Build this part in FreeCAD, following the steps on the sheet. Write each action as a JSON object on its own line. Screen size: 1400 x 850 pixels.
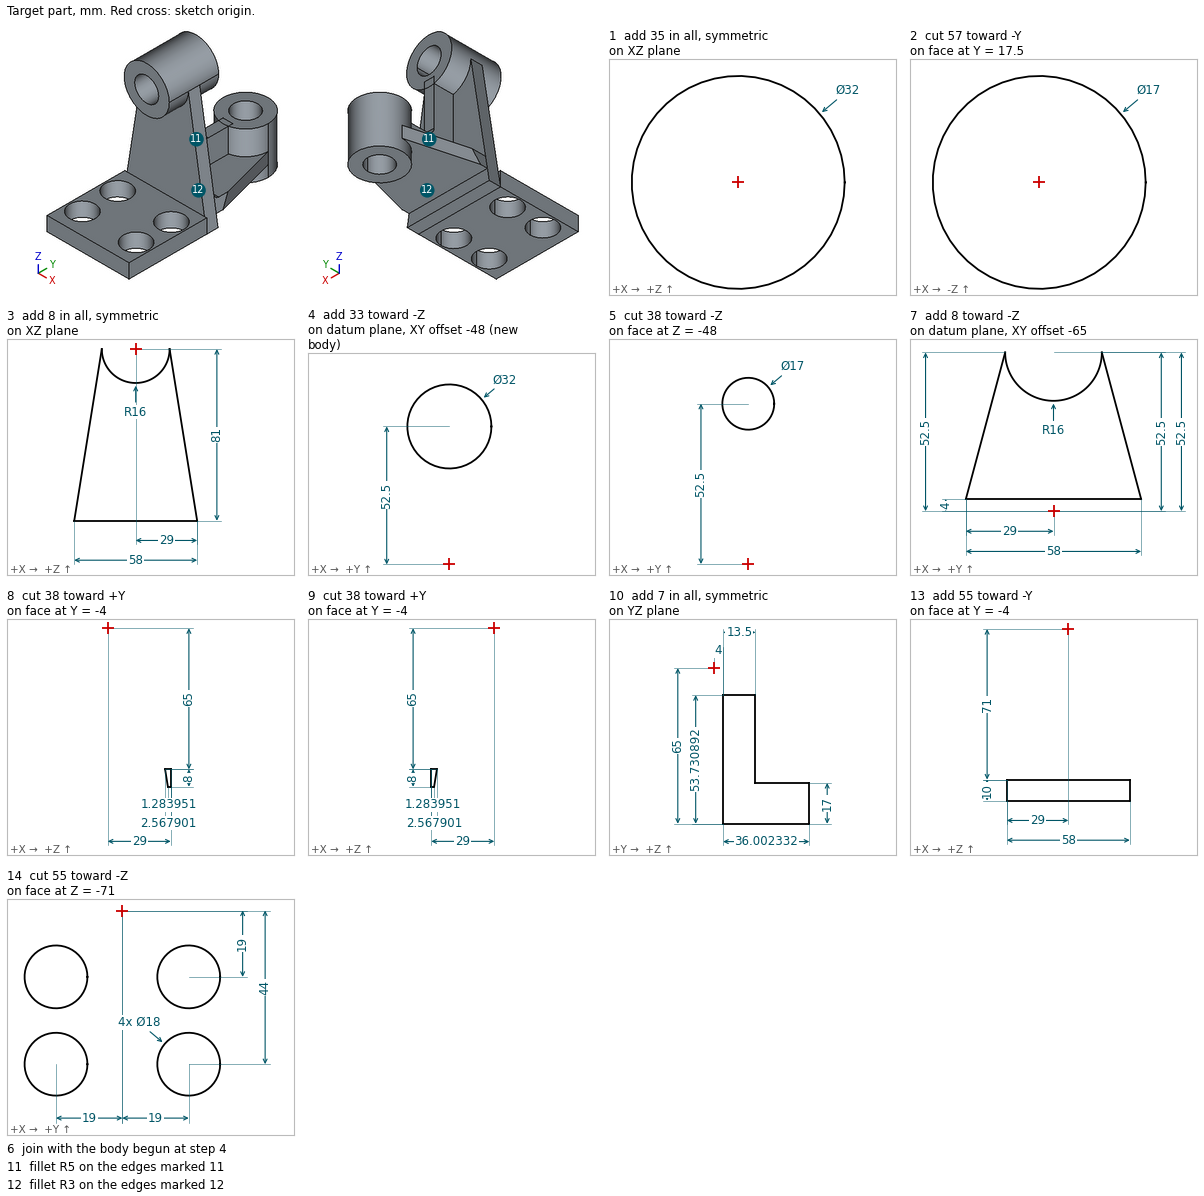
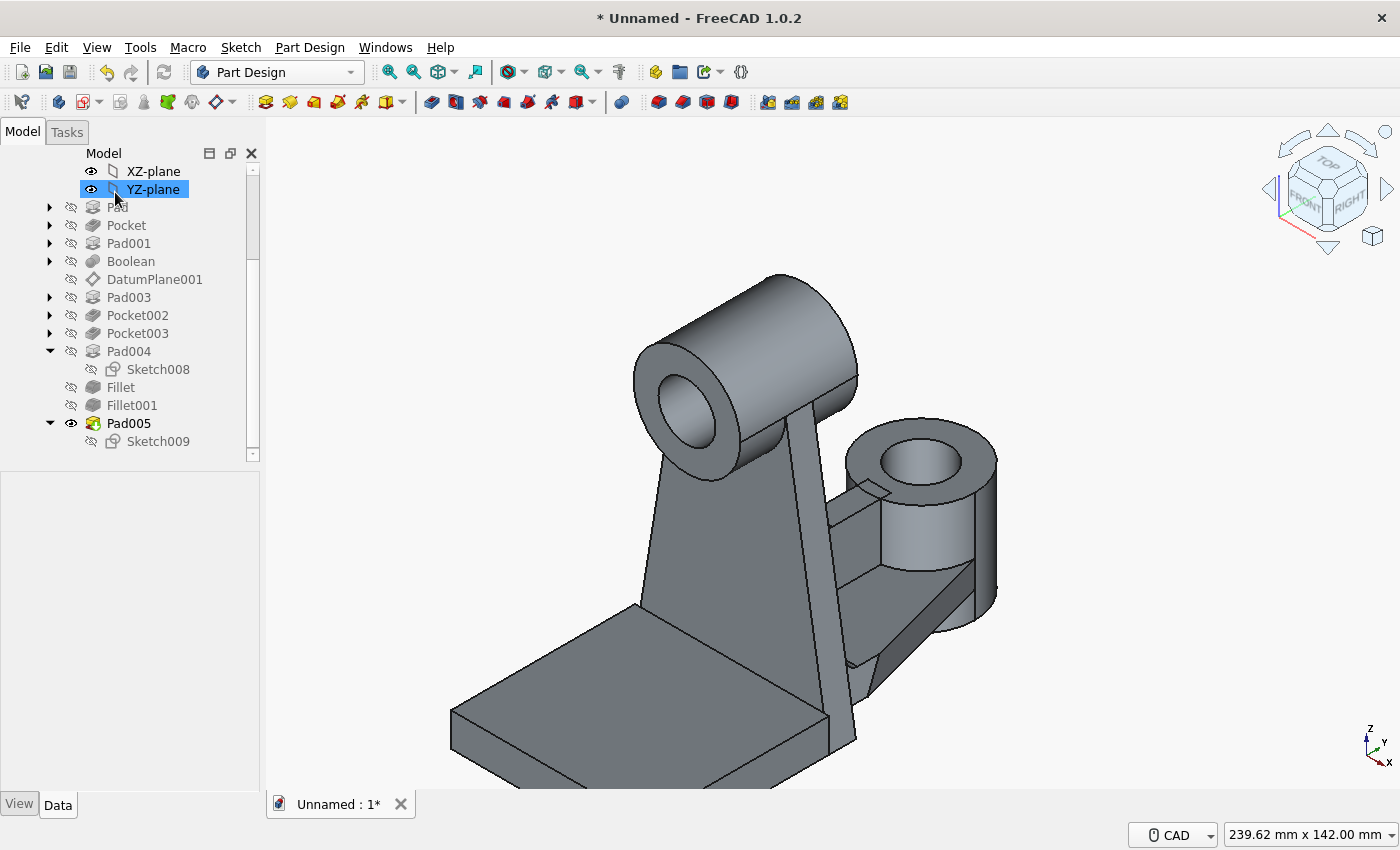
{"action": "left_click", "coordinate": [390, 72]}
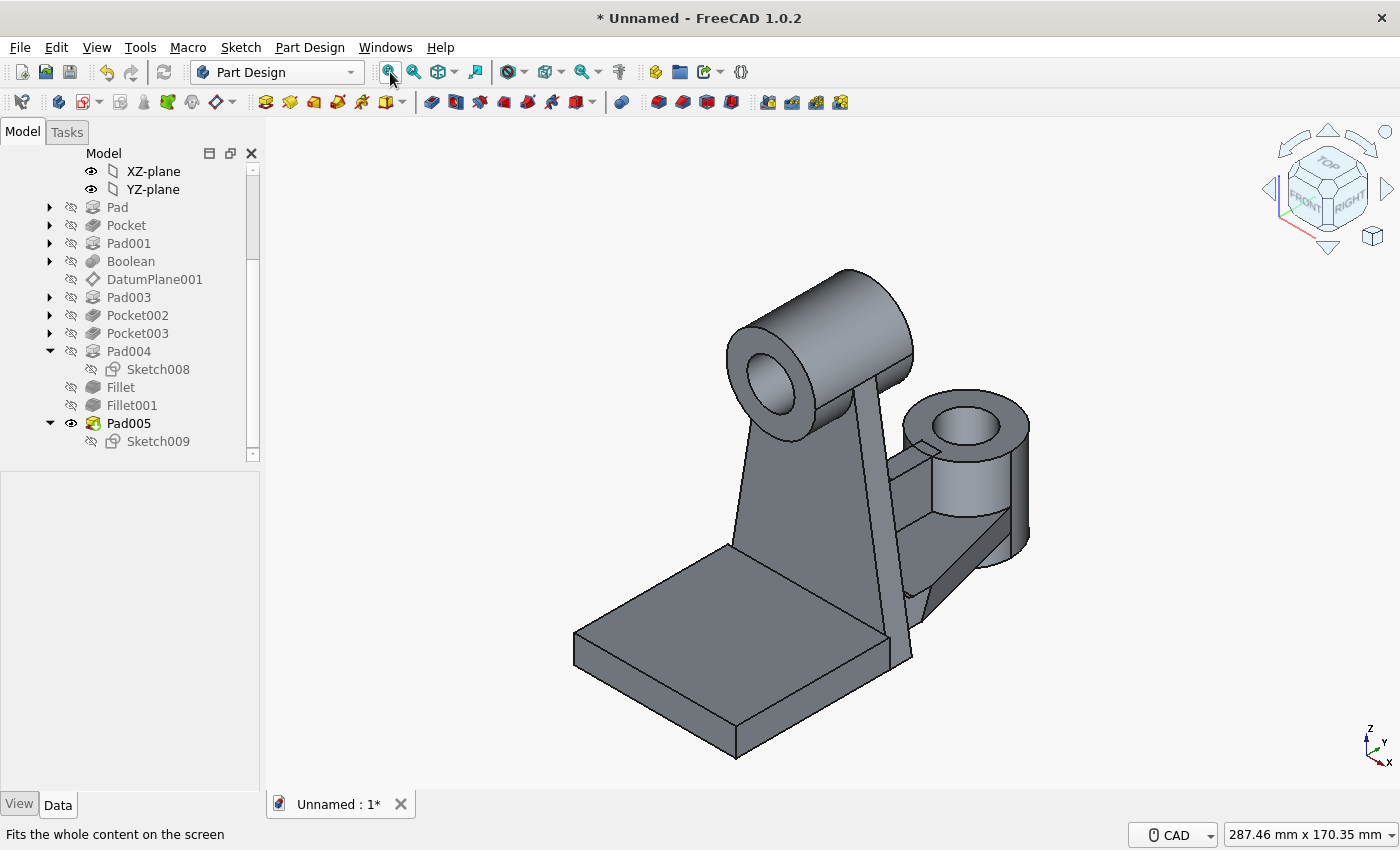
{"action": "left_click", "coordinate": [732, 634]}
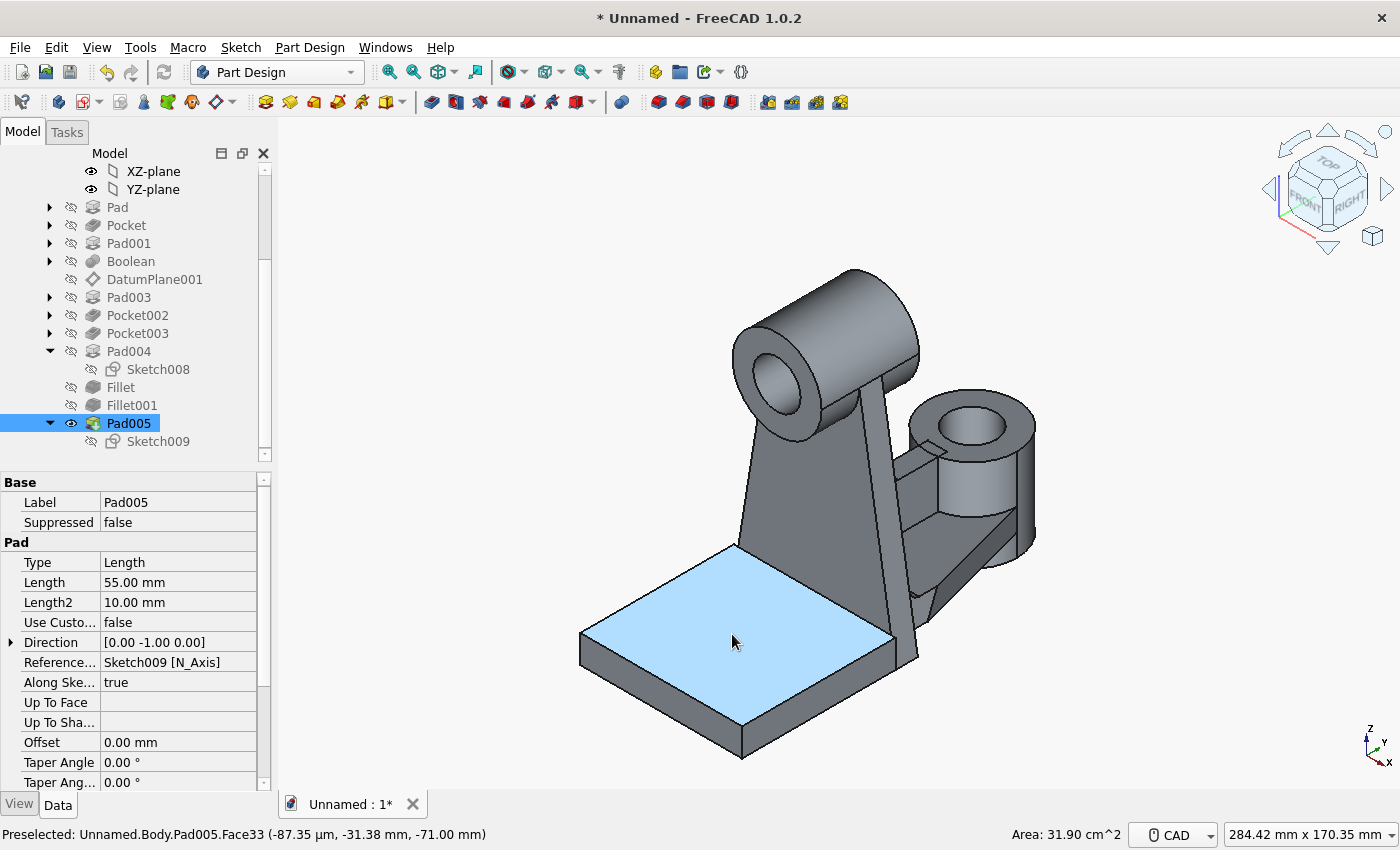
{"action": "left_click", "coordinate": [84, 102]}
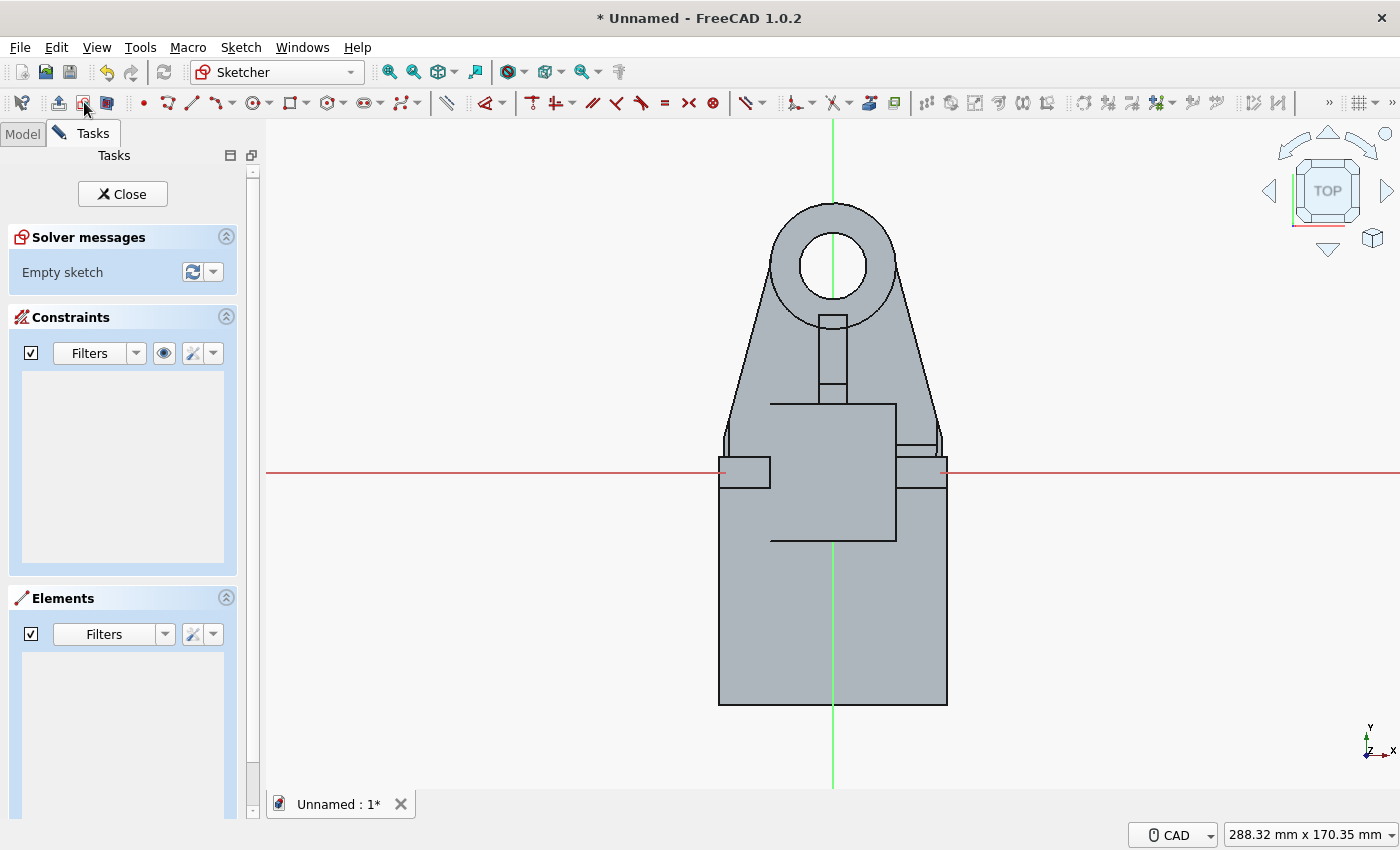
{"action": "left_click", "coordinate": [108, 104]}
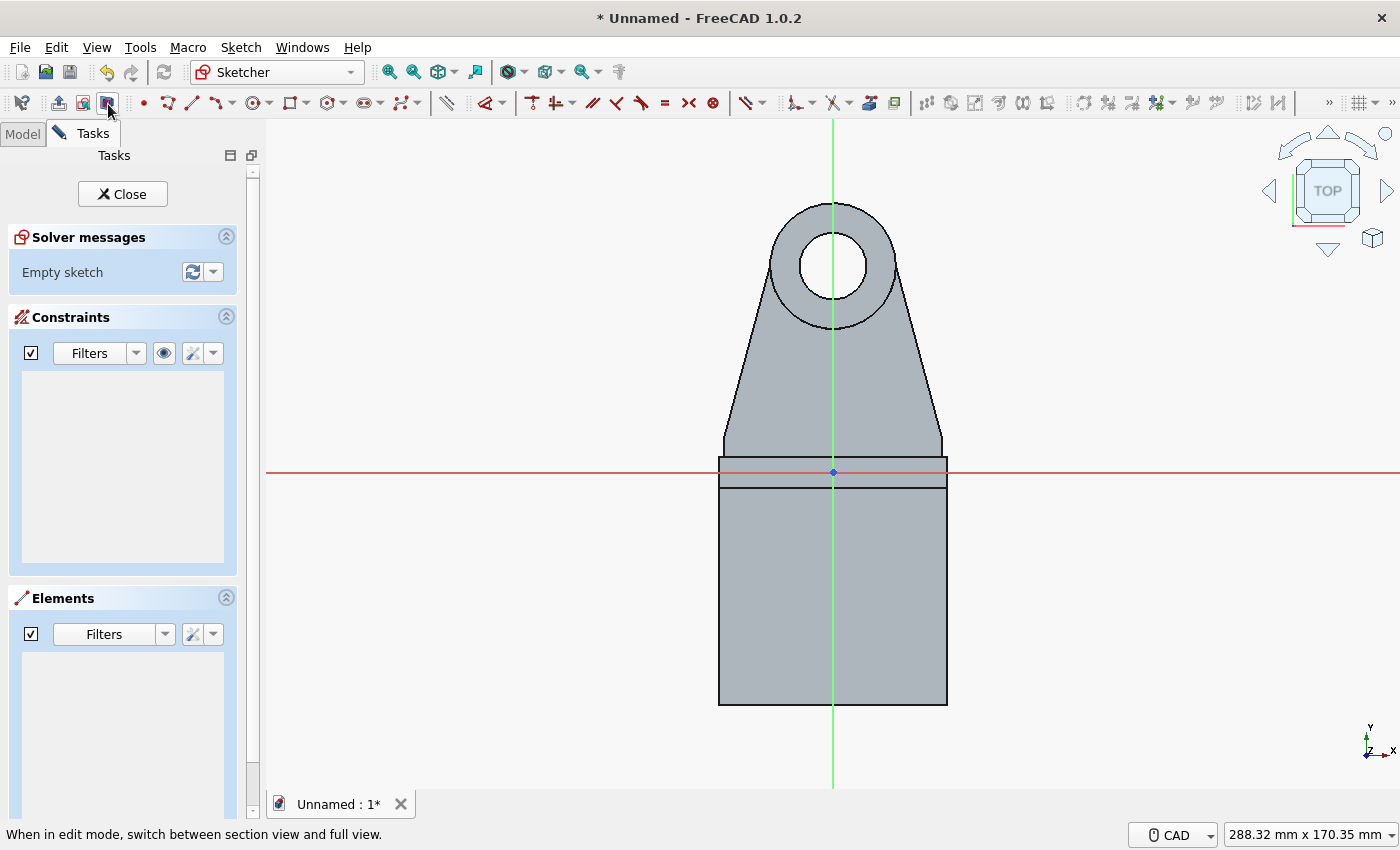
{"action": "scroll", "coordinate": [889, 677], "scroll_direction": "up", "scroll_amount": 4}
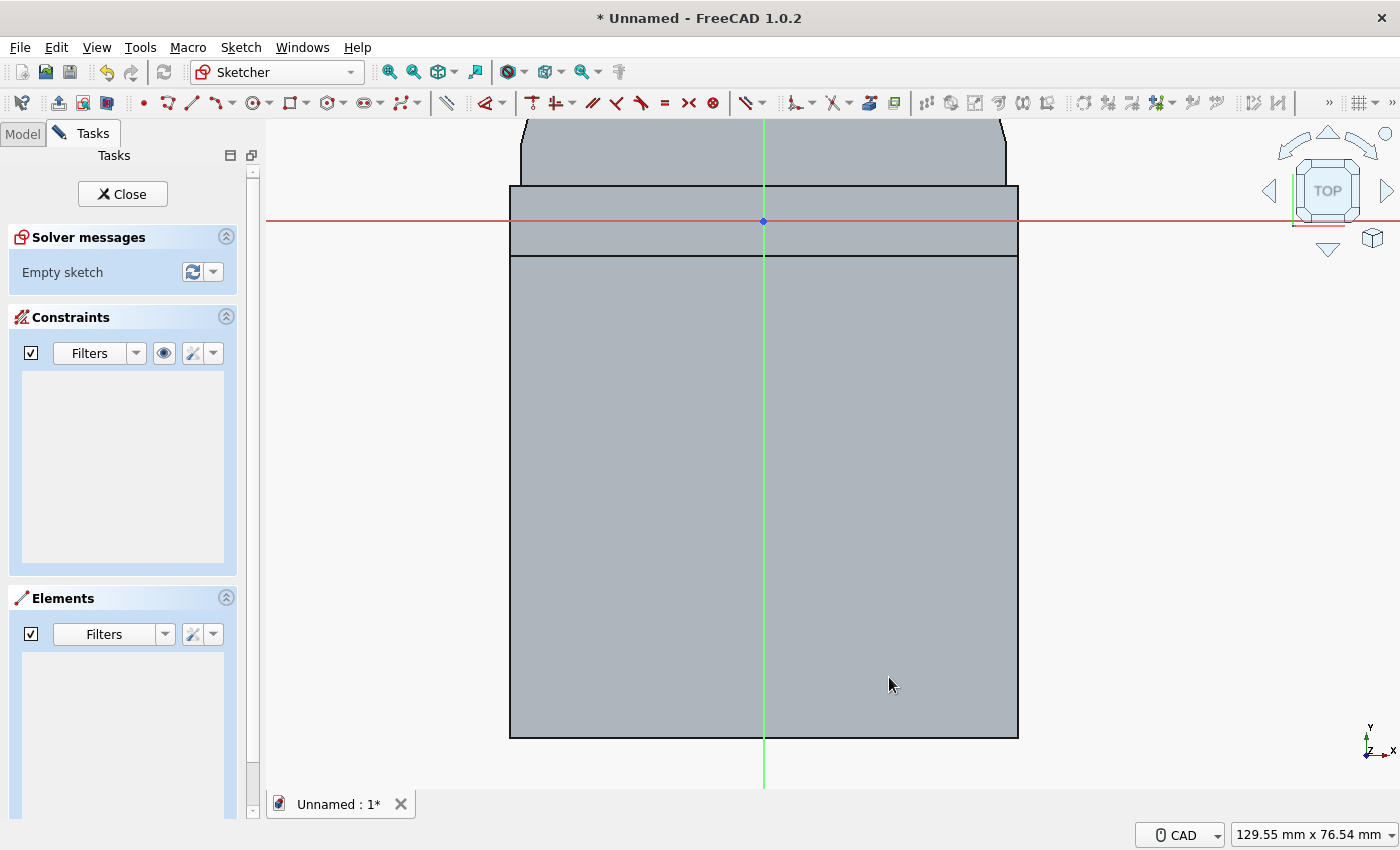
{"action": "key", "text": "g c"}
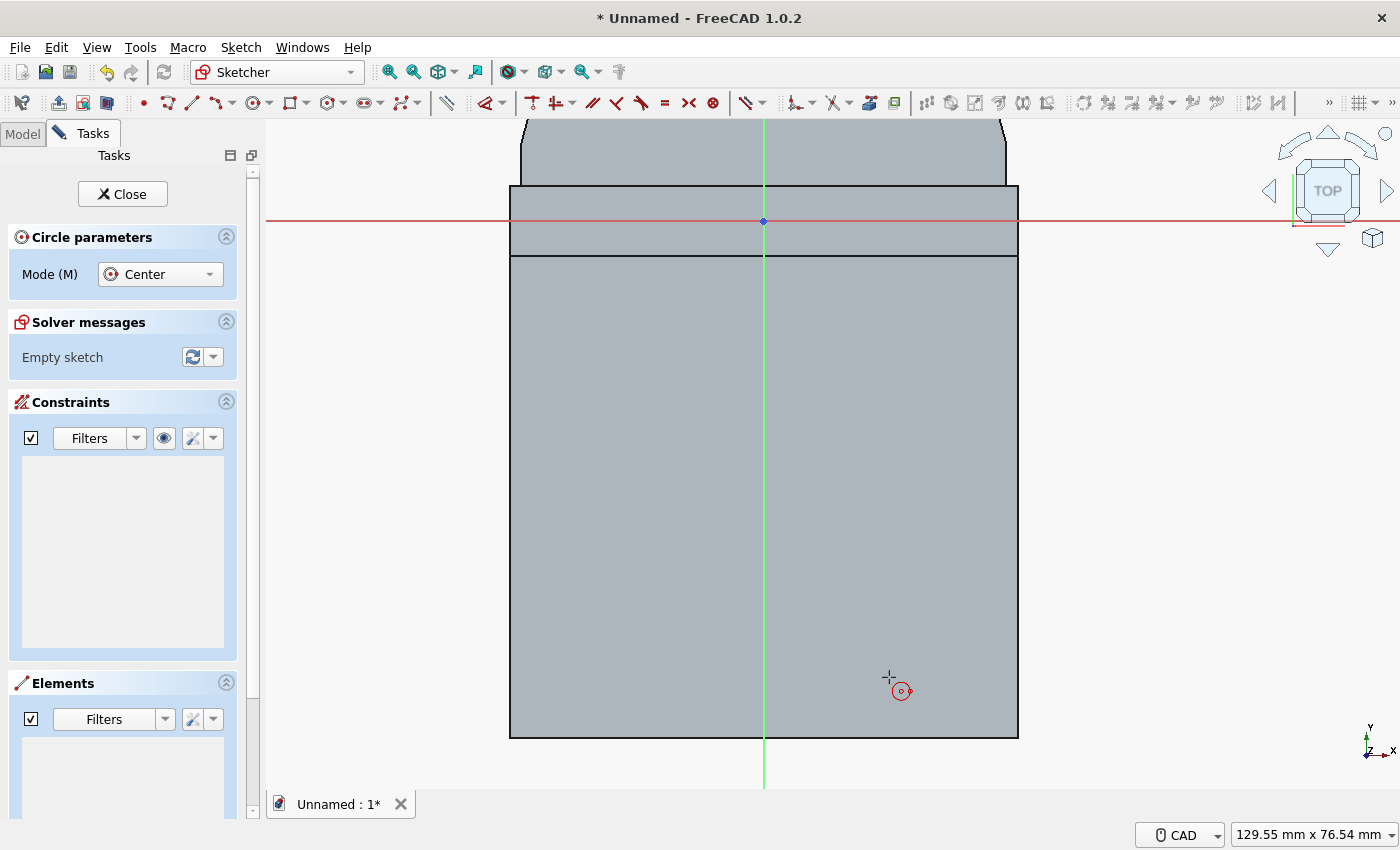
{"action": "left_click", "coordinate": [930, 606]}
{"action": "left_click", "coordinate": [986, 551]}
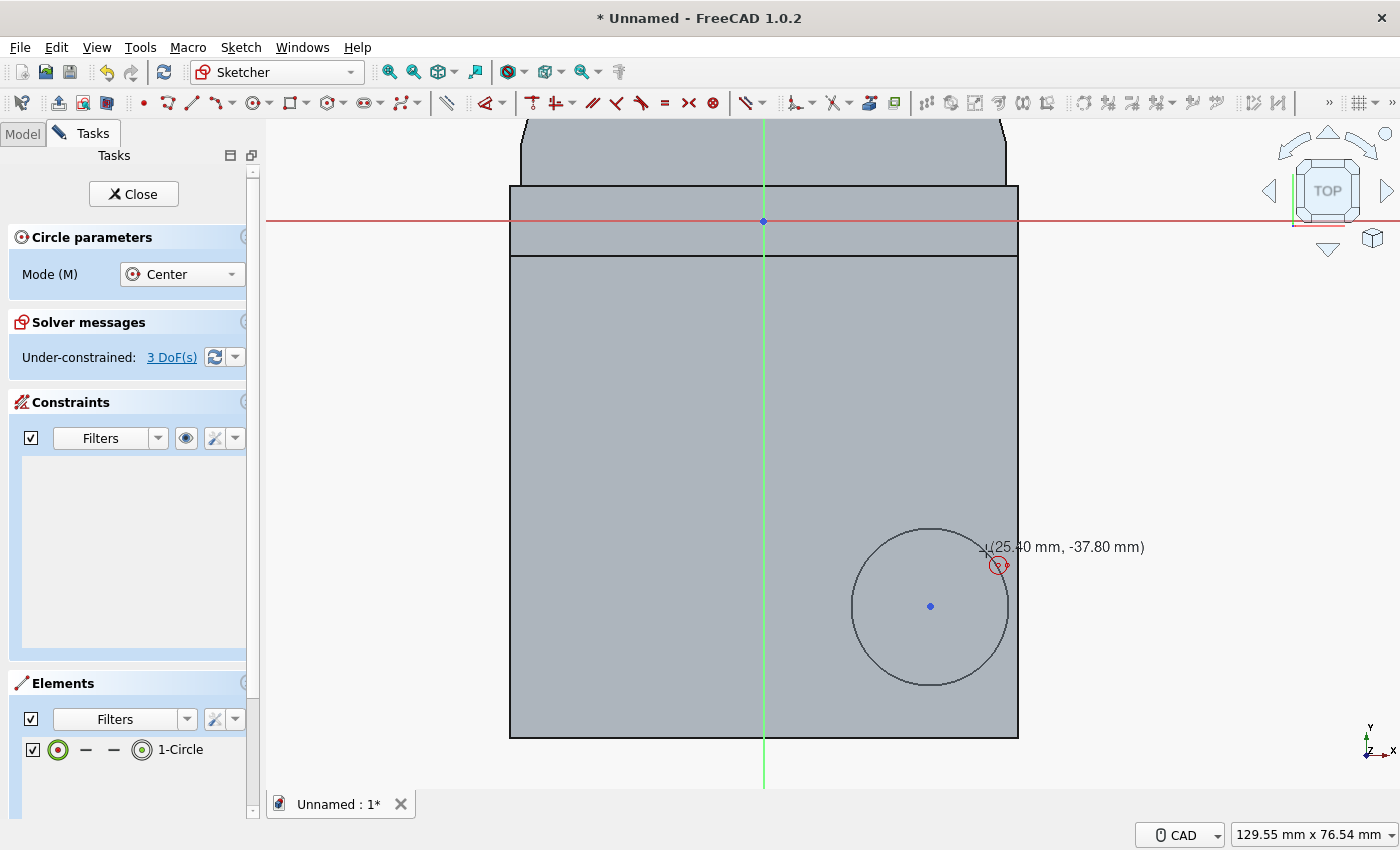
{"action": "left_click", "coordinate": [930, 387]}
{"action": "left_click", "coordinate": [986, 332]}